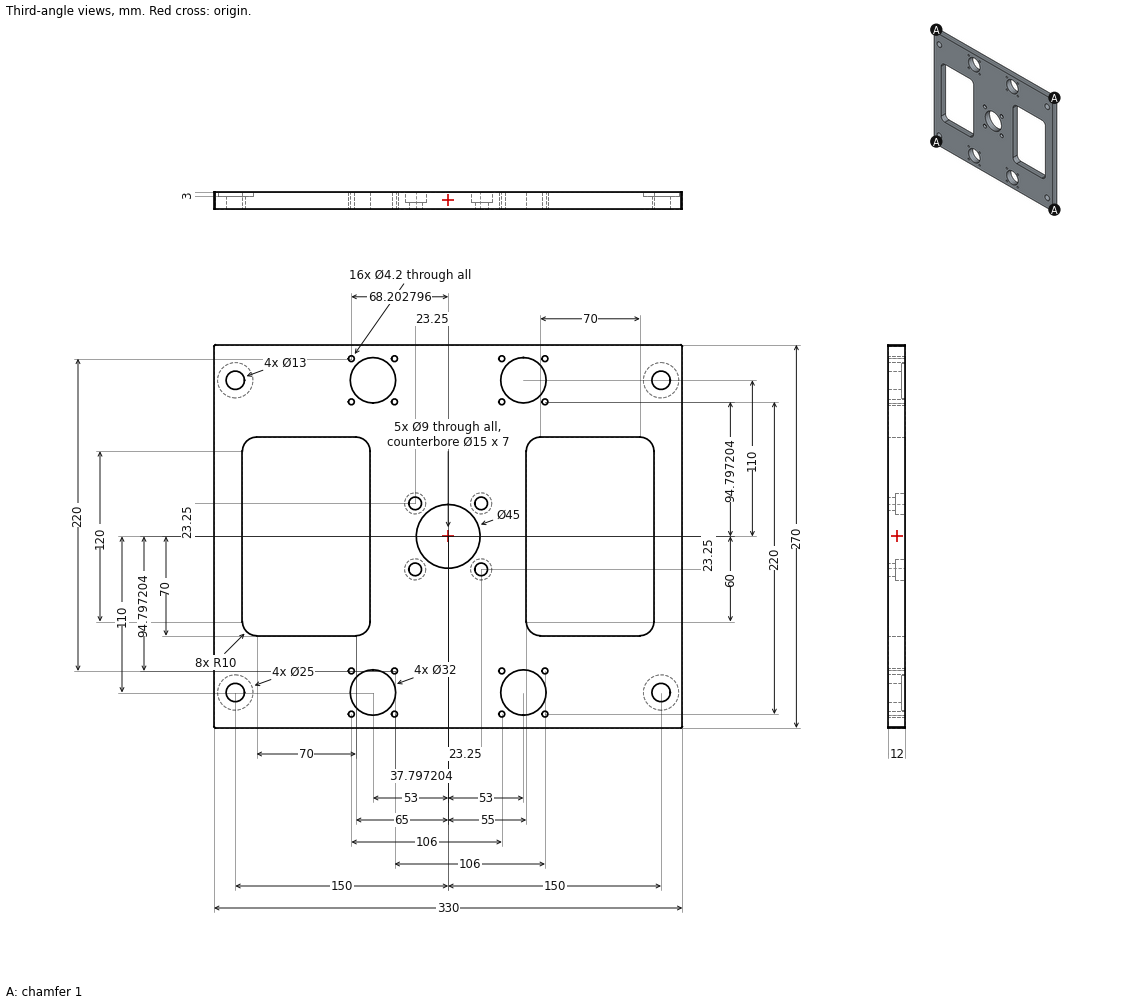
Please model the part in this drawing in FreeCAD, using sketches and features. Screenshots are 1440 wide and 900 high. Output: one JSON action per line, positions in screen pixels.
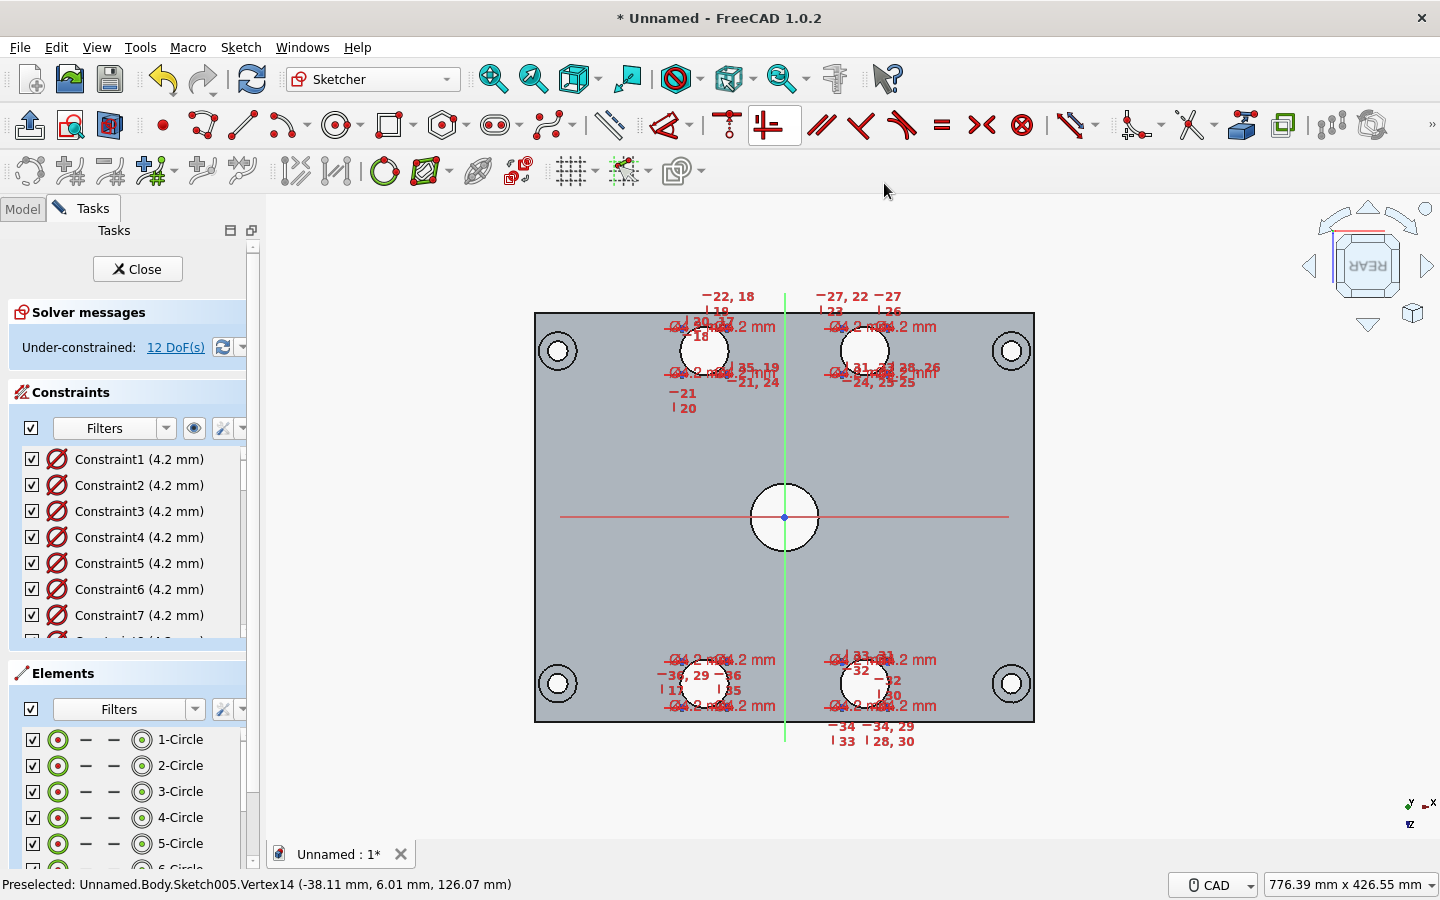
{"action": "left_click", "coordinate": [727, 708]}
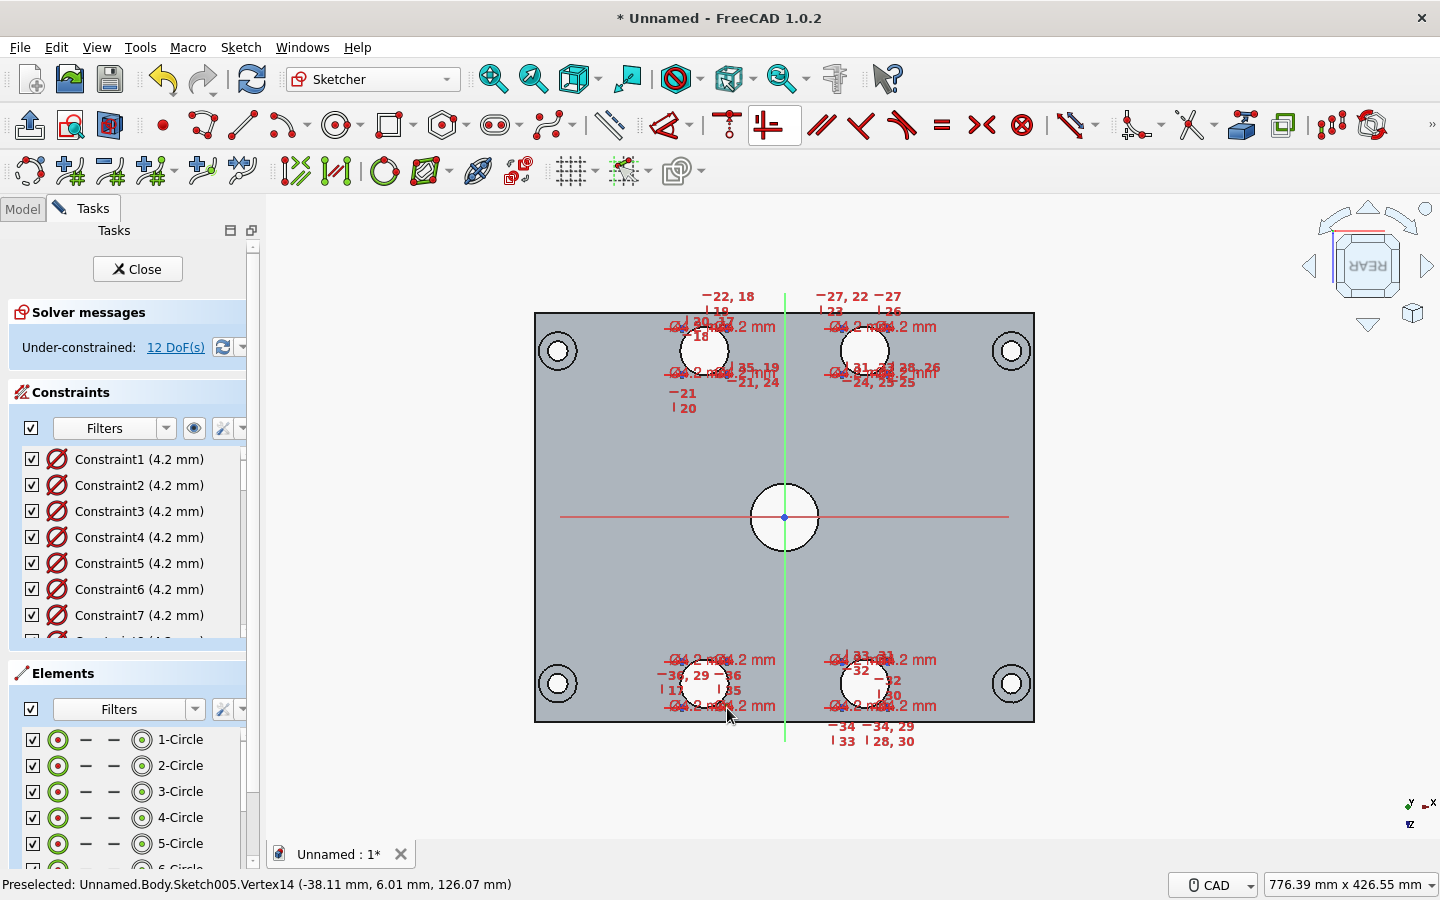
{"action": "left_click", "coordinate": [727, 662]}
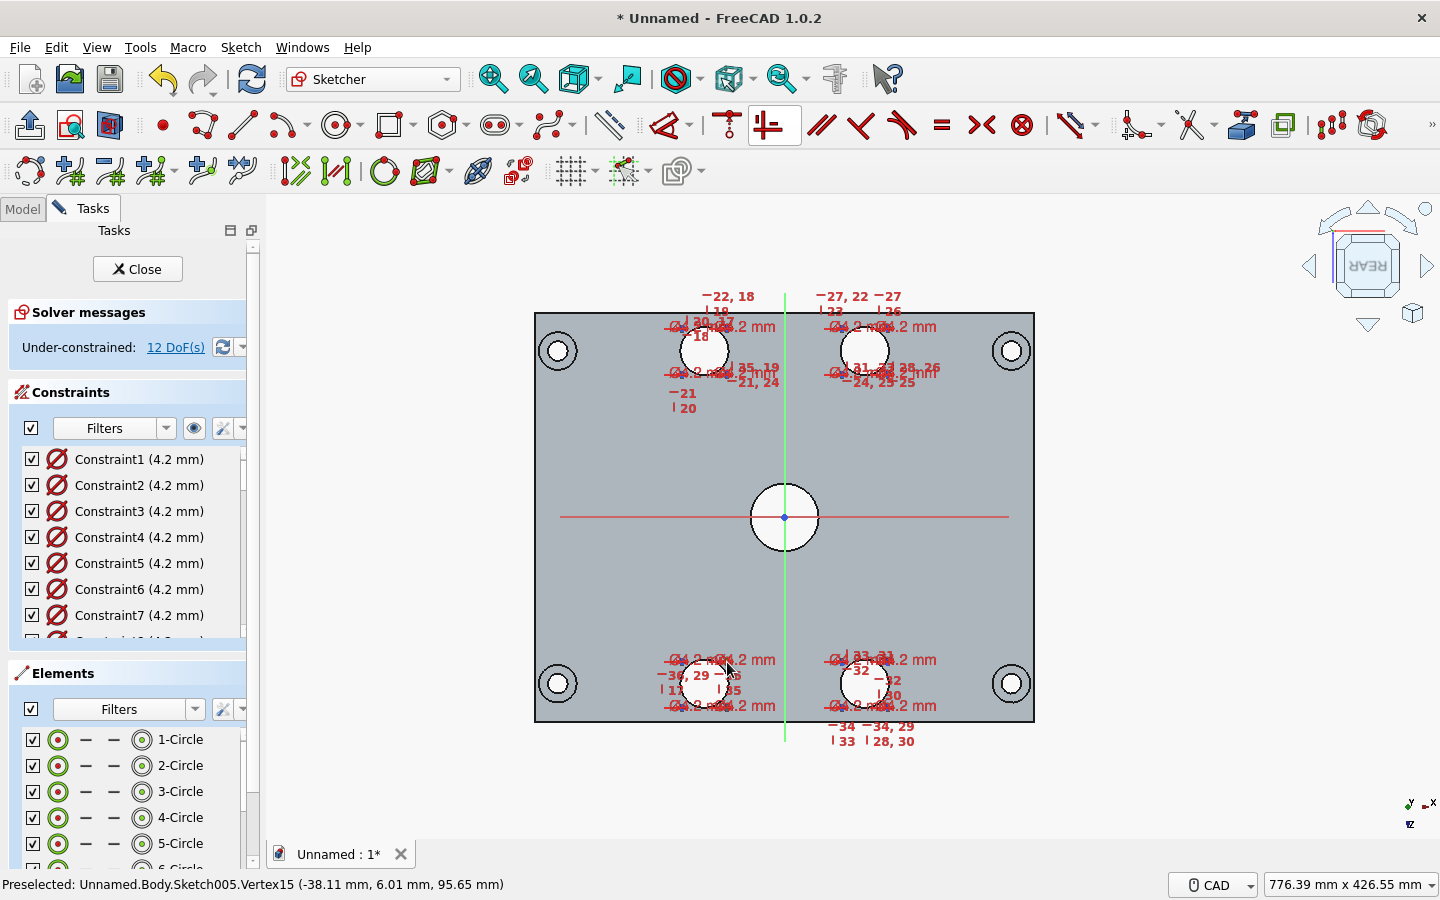
{"action": "key", "text": "v"}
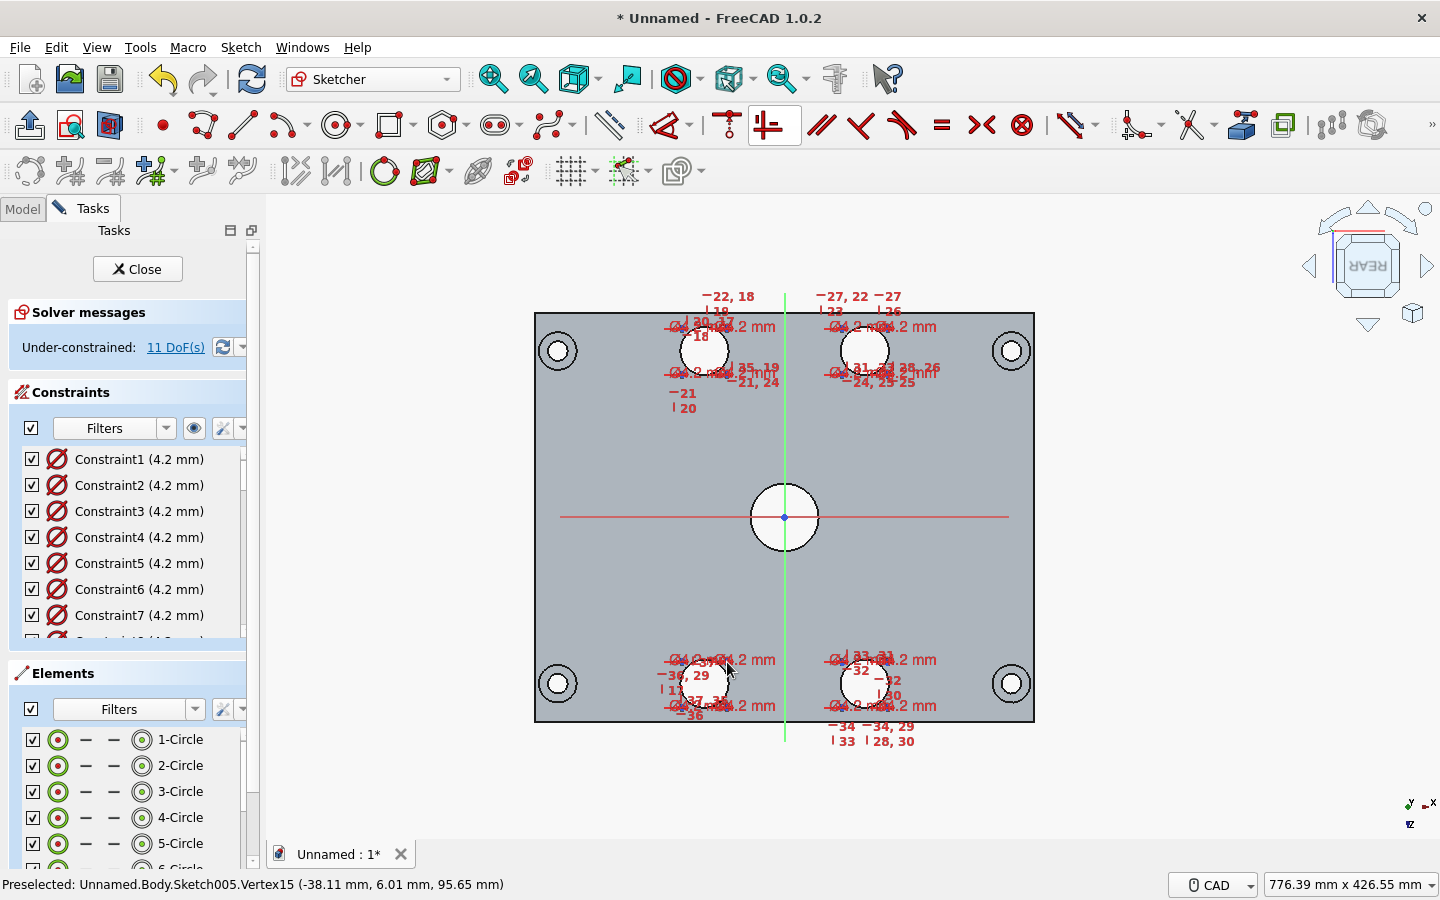
{"action": "left_click", "coordinate": [842, 662]}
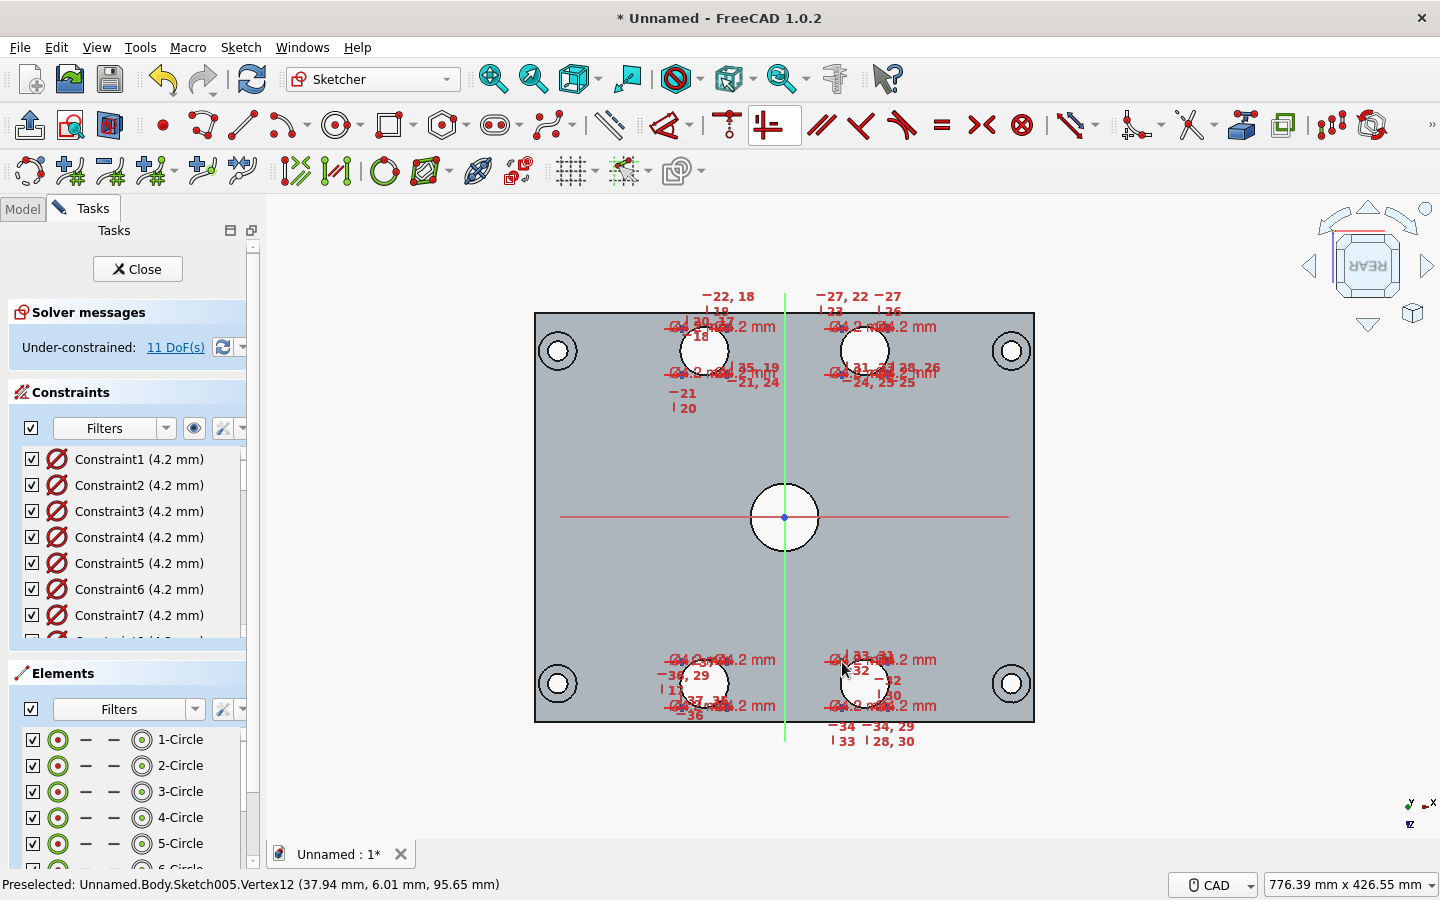
{"action": "left_click", "coordinate": [727, 662]}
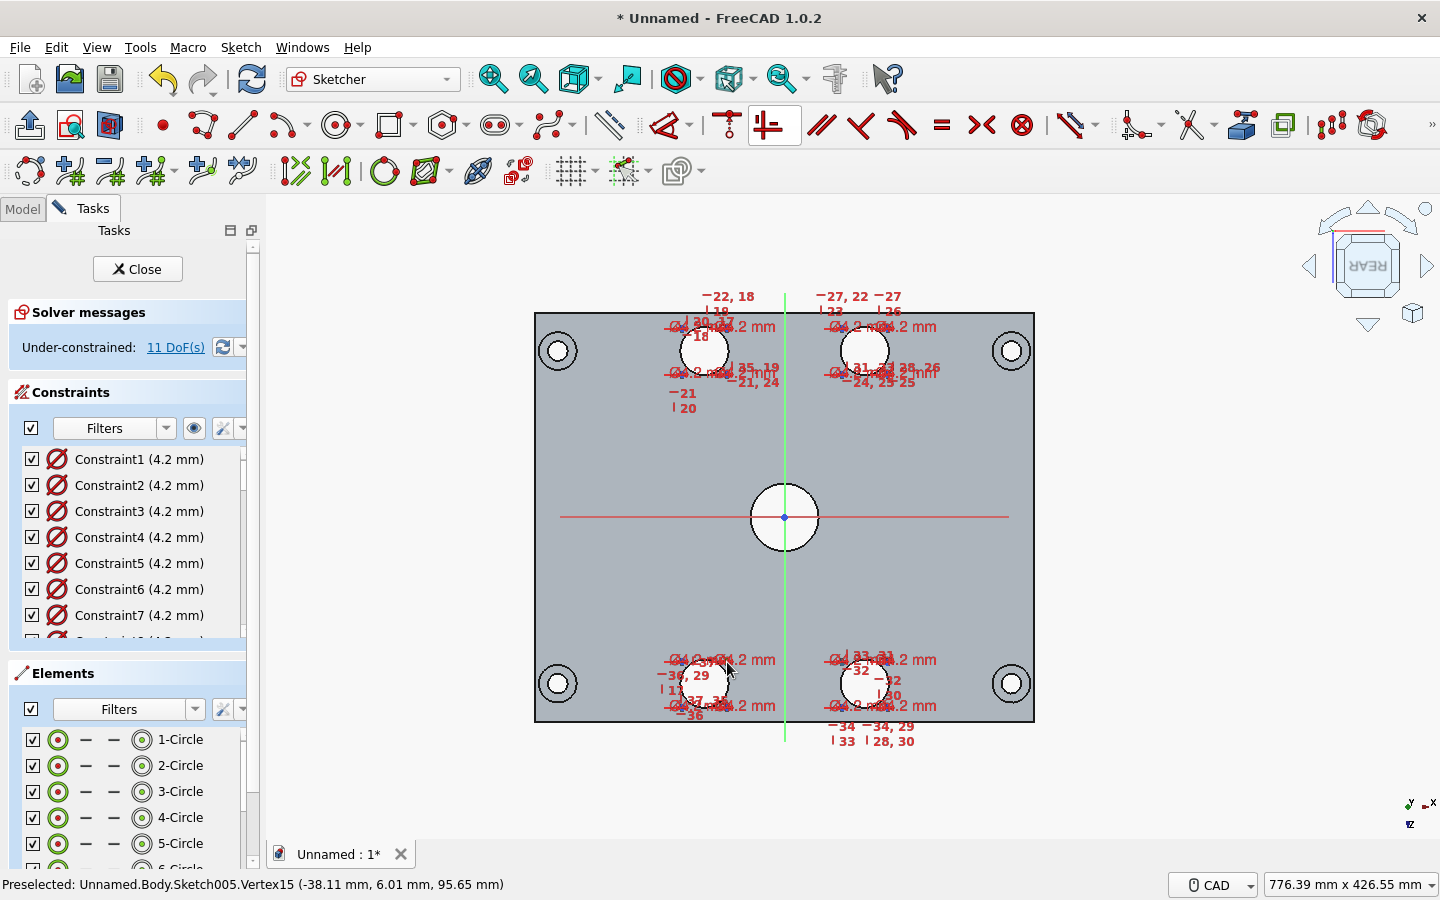
{"action": "left_click", "coordinate": [796, 126]}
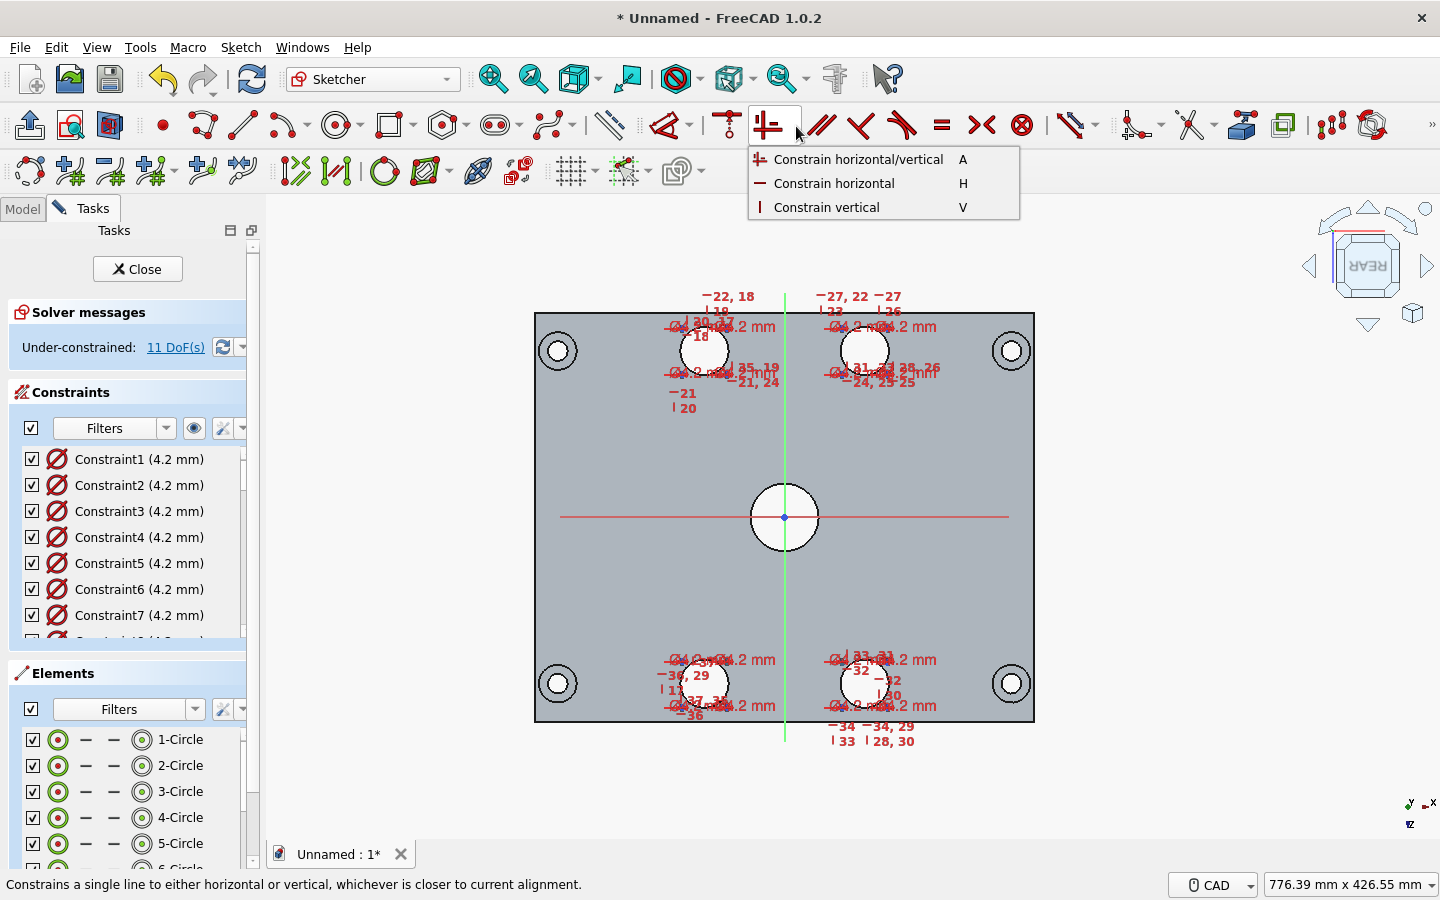
{"action": "left_click", "coordinate": [884, 183]}